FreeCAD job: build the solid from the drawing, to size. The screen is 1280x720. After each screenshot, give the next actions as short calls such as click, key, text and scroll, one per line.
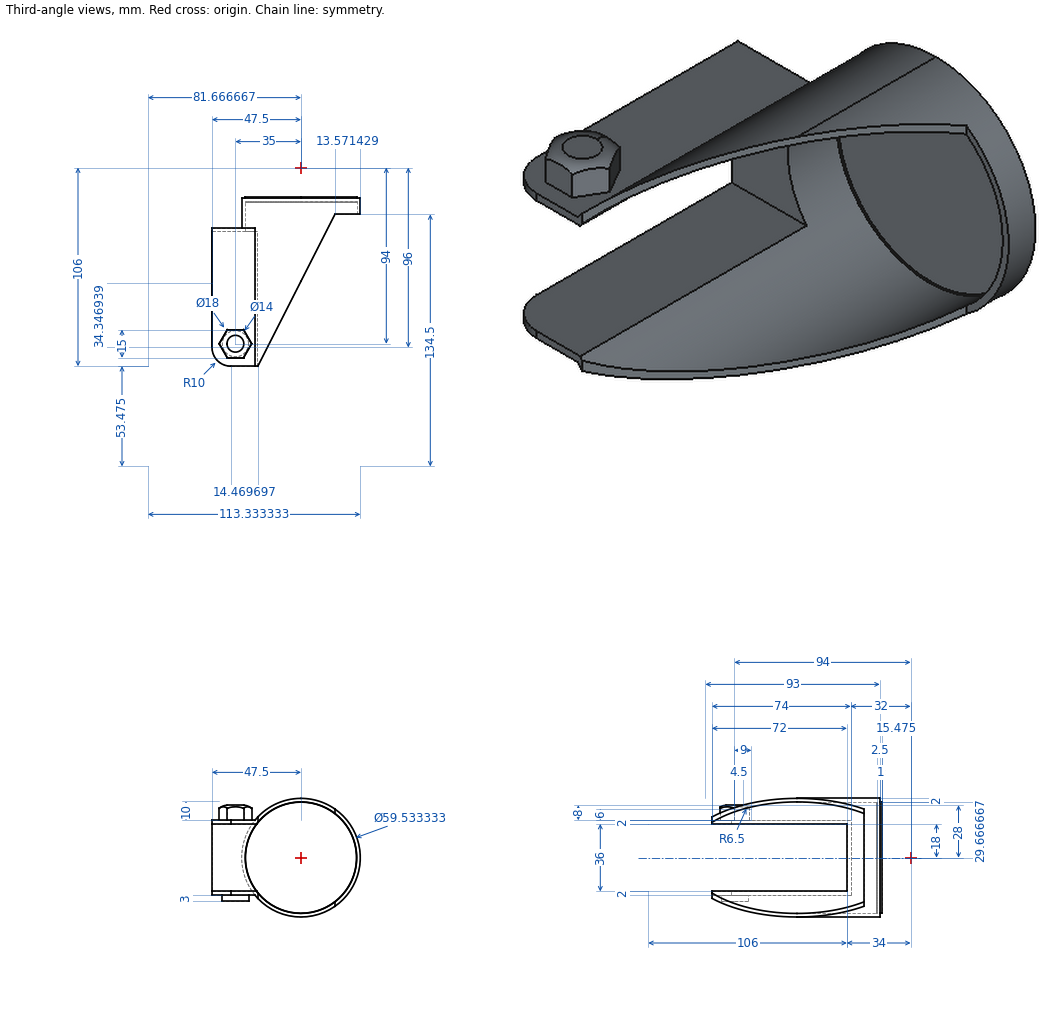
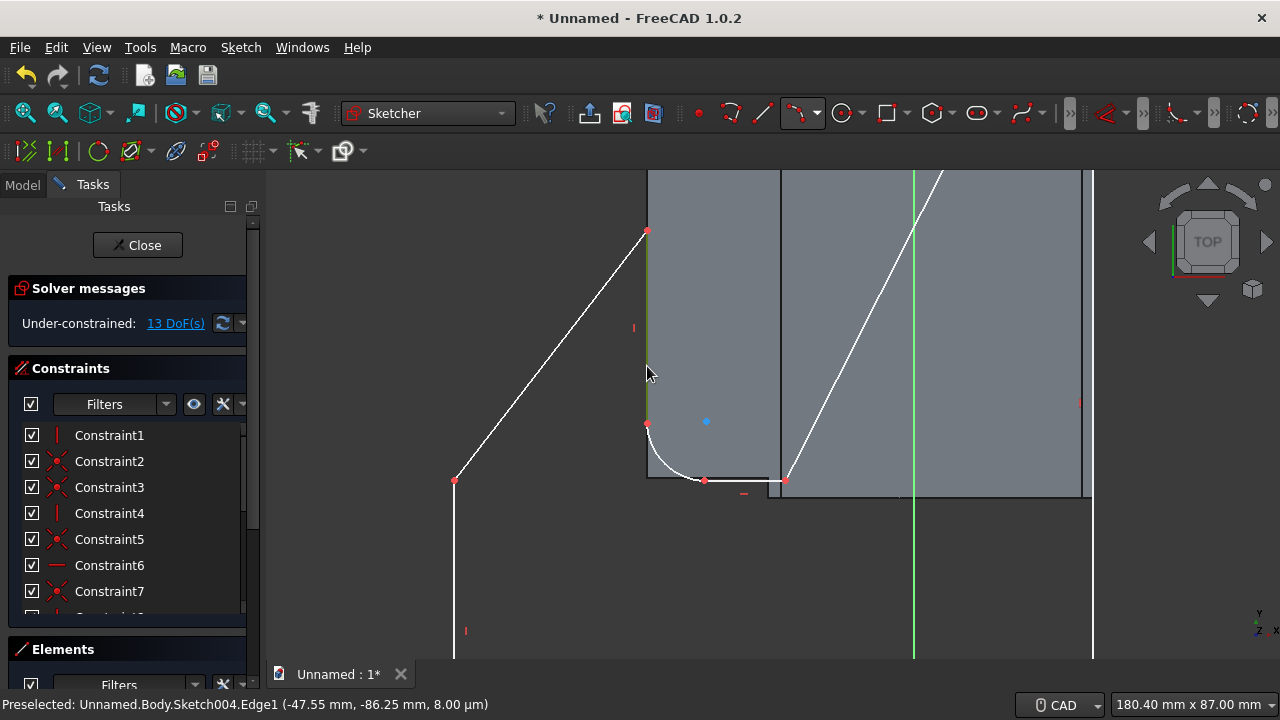
click(654, 449)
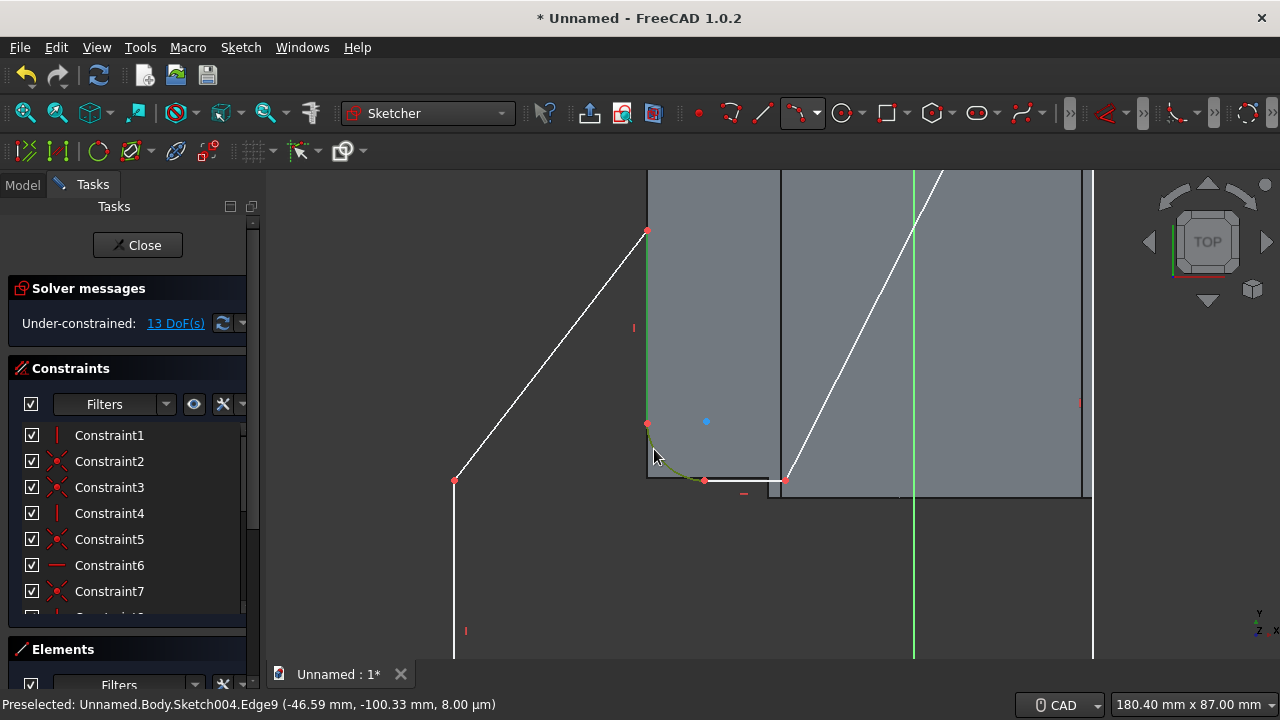
key(t)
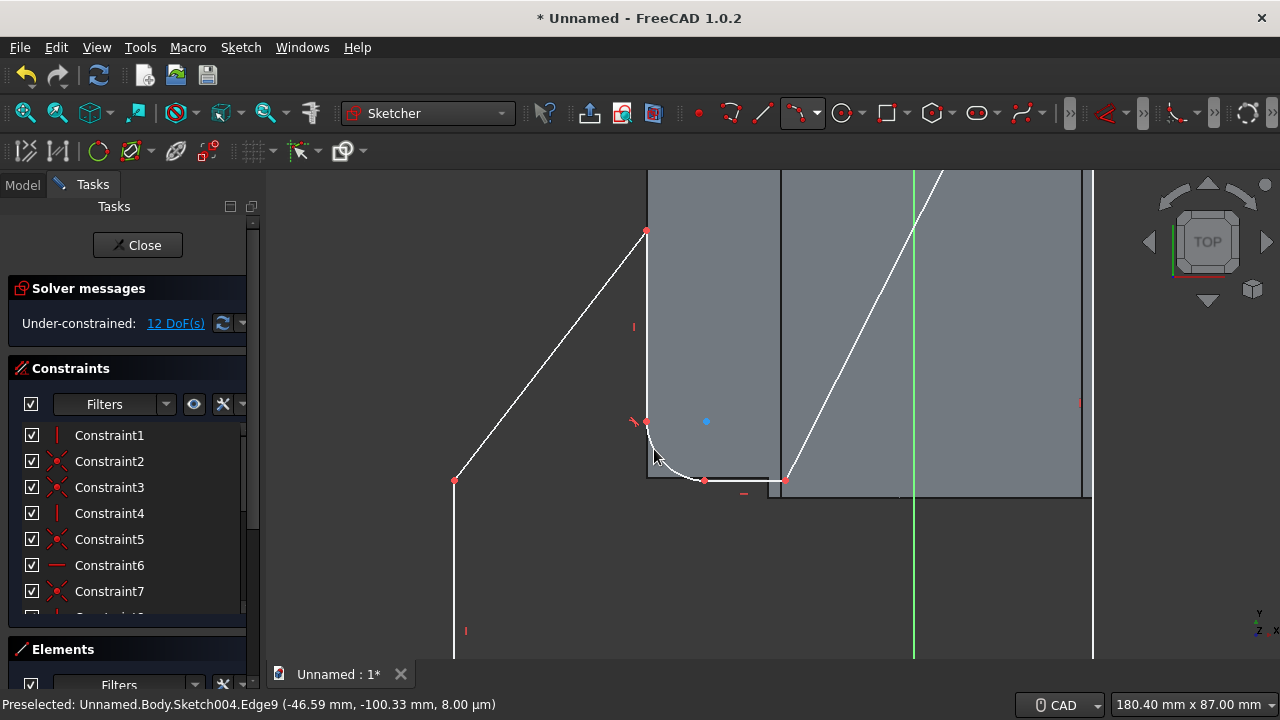
click(761, 481)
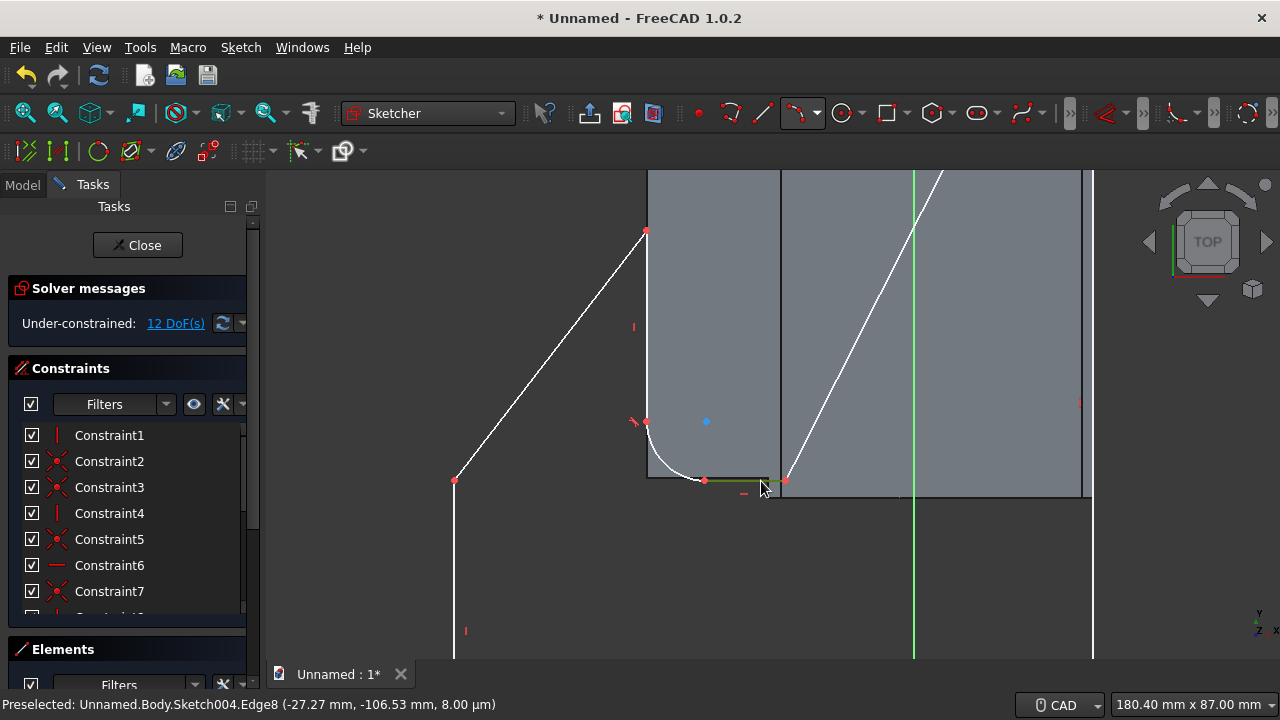
click(653, 448)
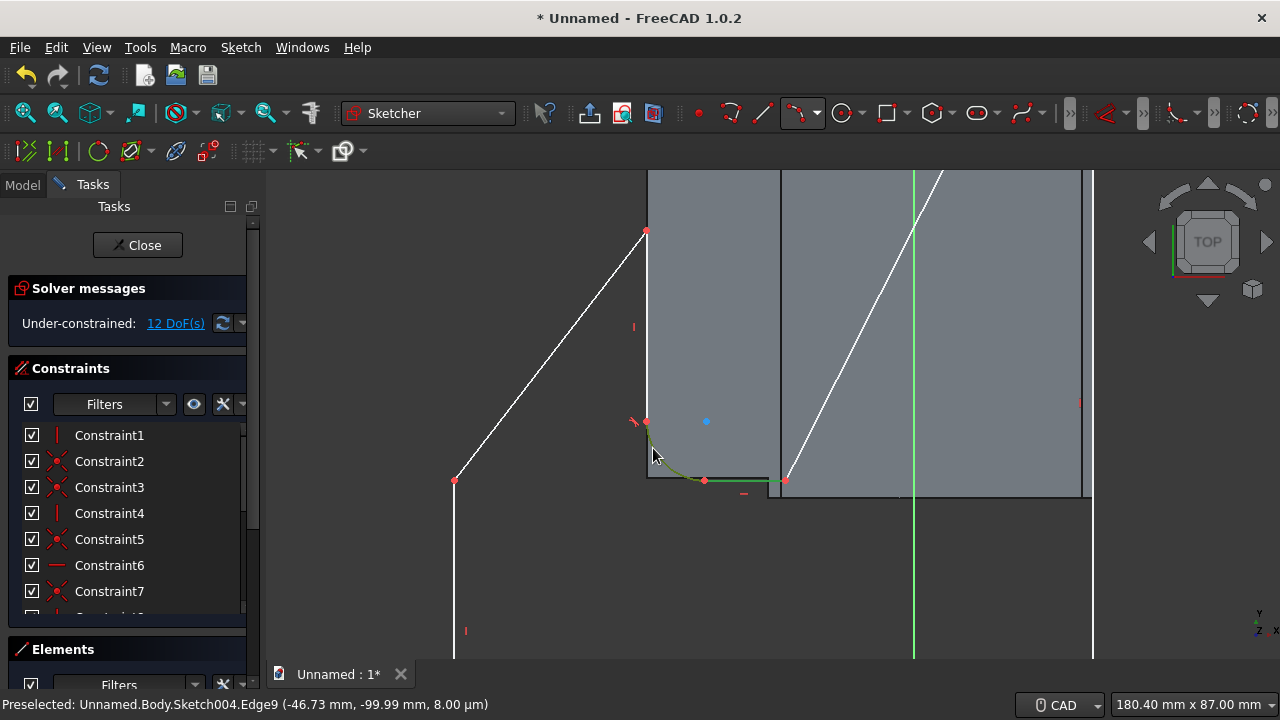
key(t)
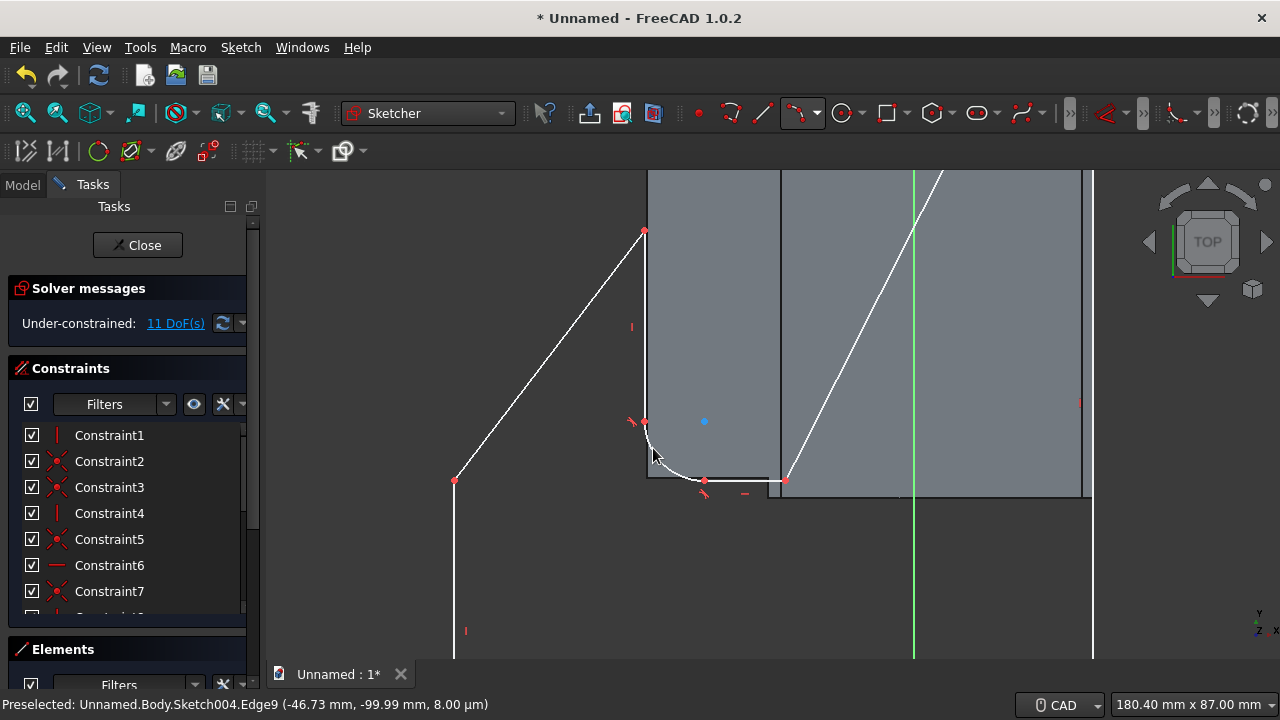
key(d)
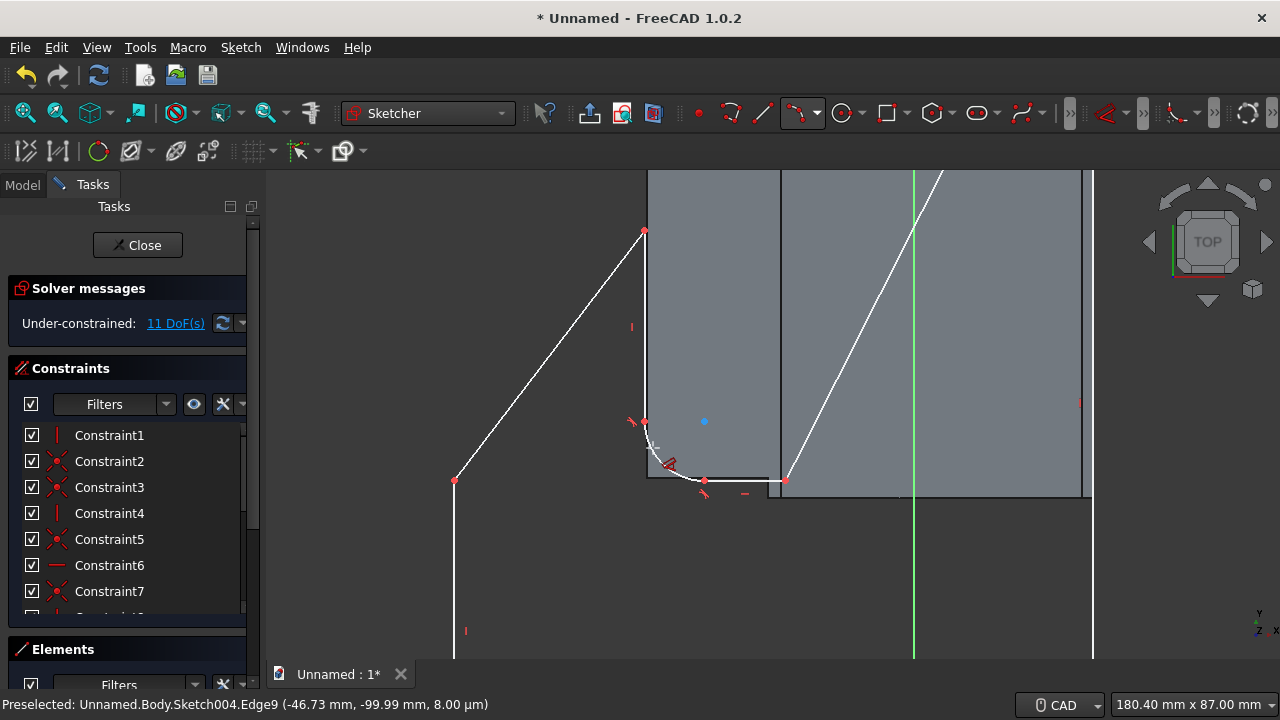
click(651, 448)
click(622, 462)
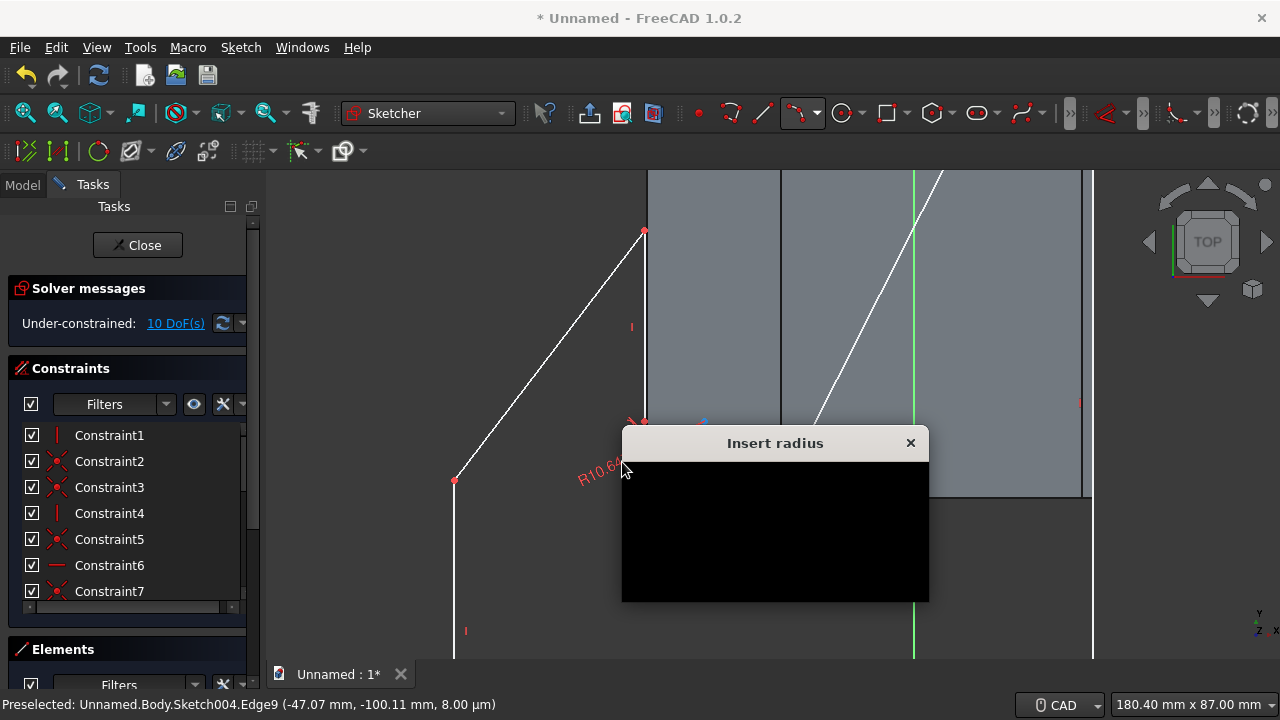
text(10)
key(Return)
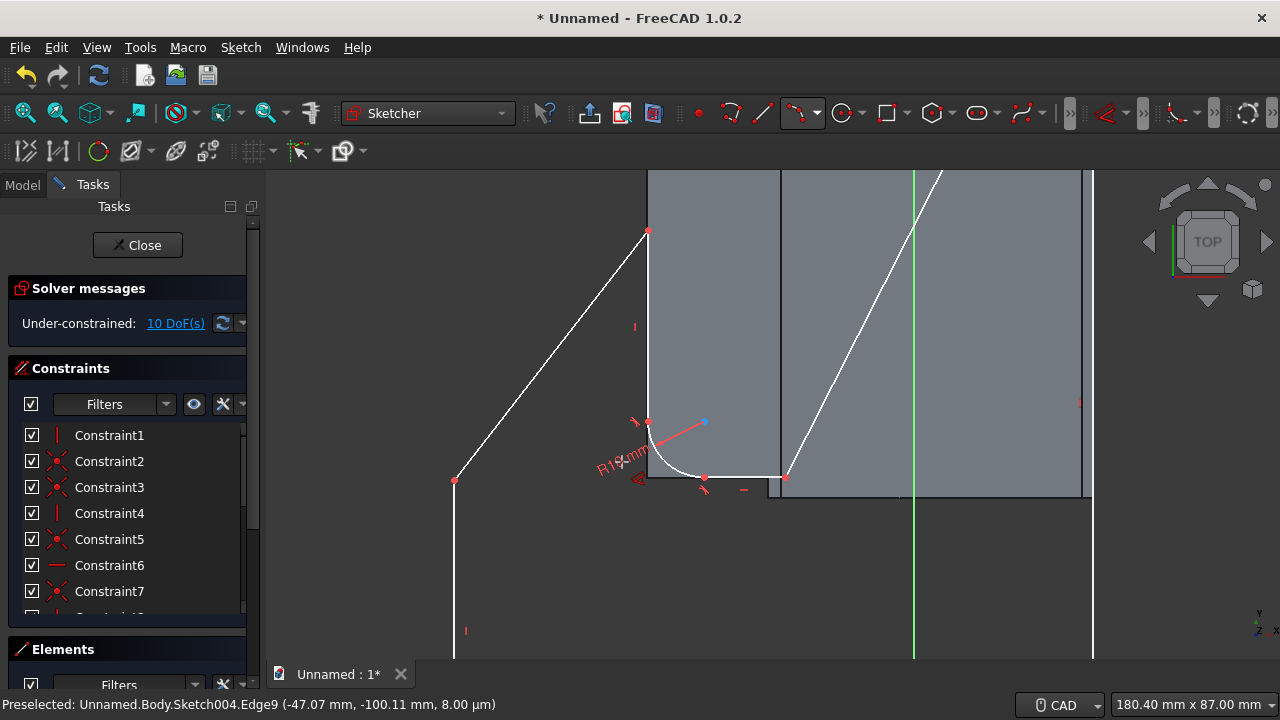
click(648, 421)
click(948, 310)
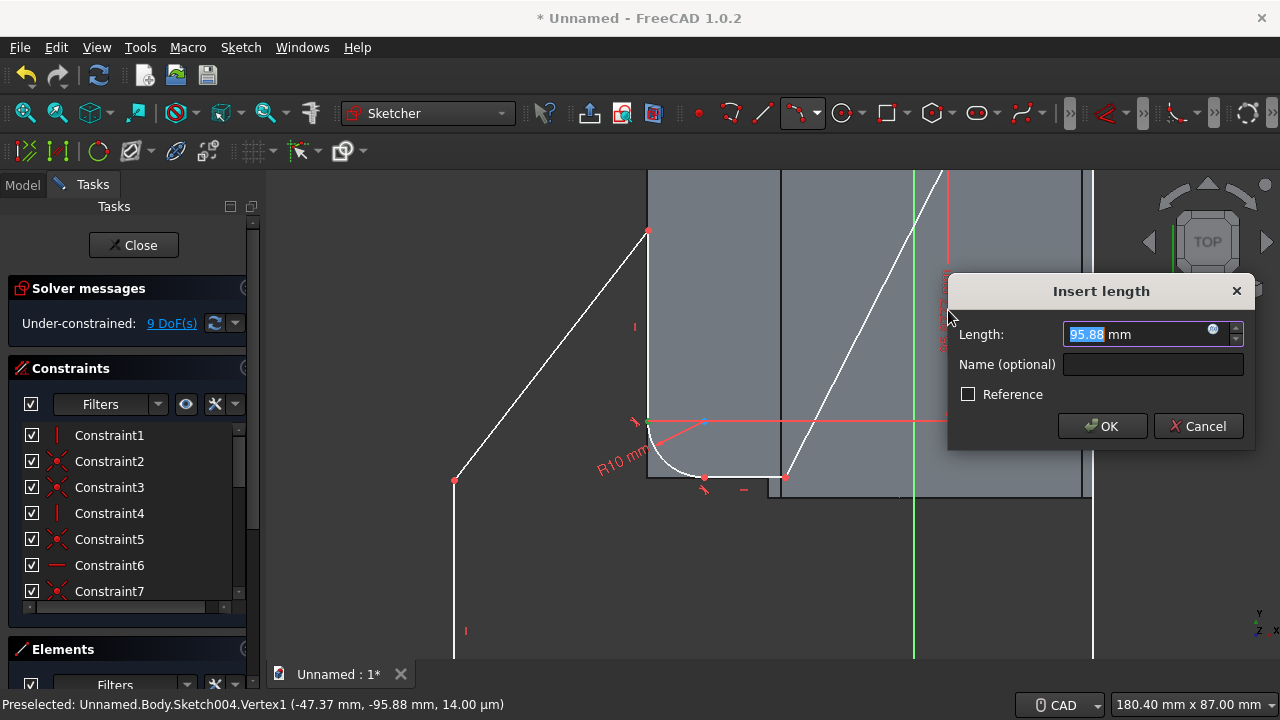
text(96)
key(Return)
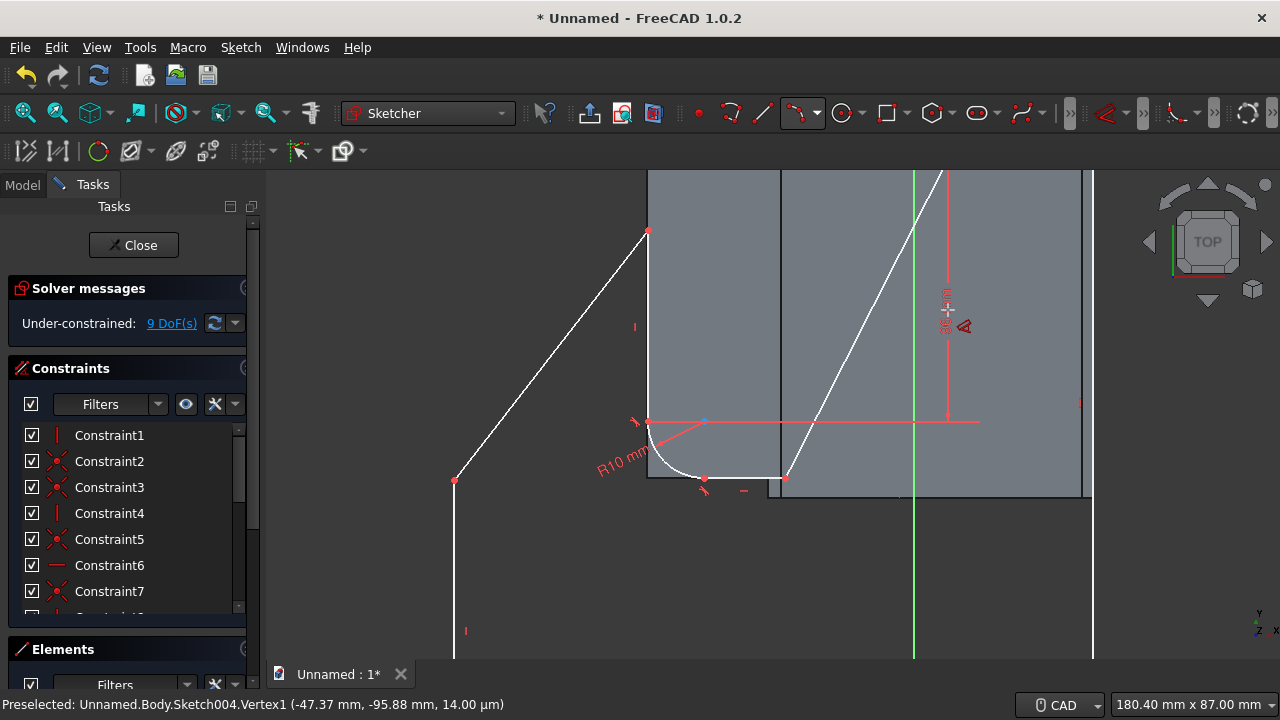
click(454, 481)
click(420, 339)